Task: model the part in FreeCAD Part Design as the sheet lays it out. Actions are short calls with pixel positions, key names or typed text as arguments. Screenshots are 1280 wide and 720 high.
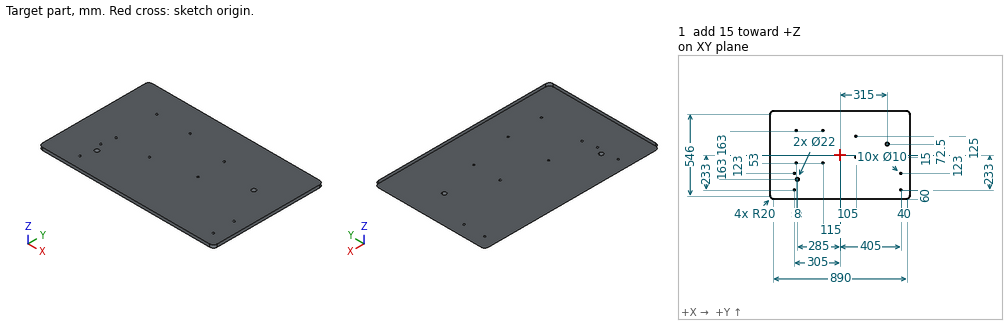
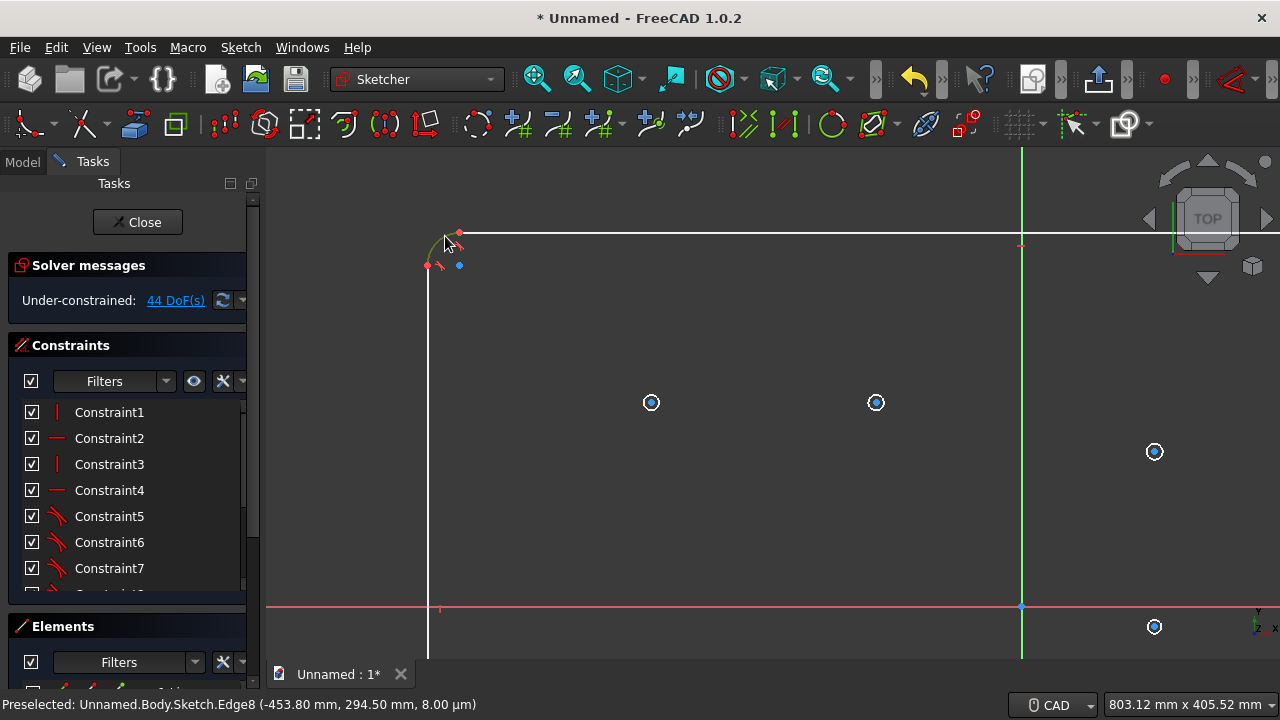
key(e)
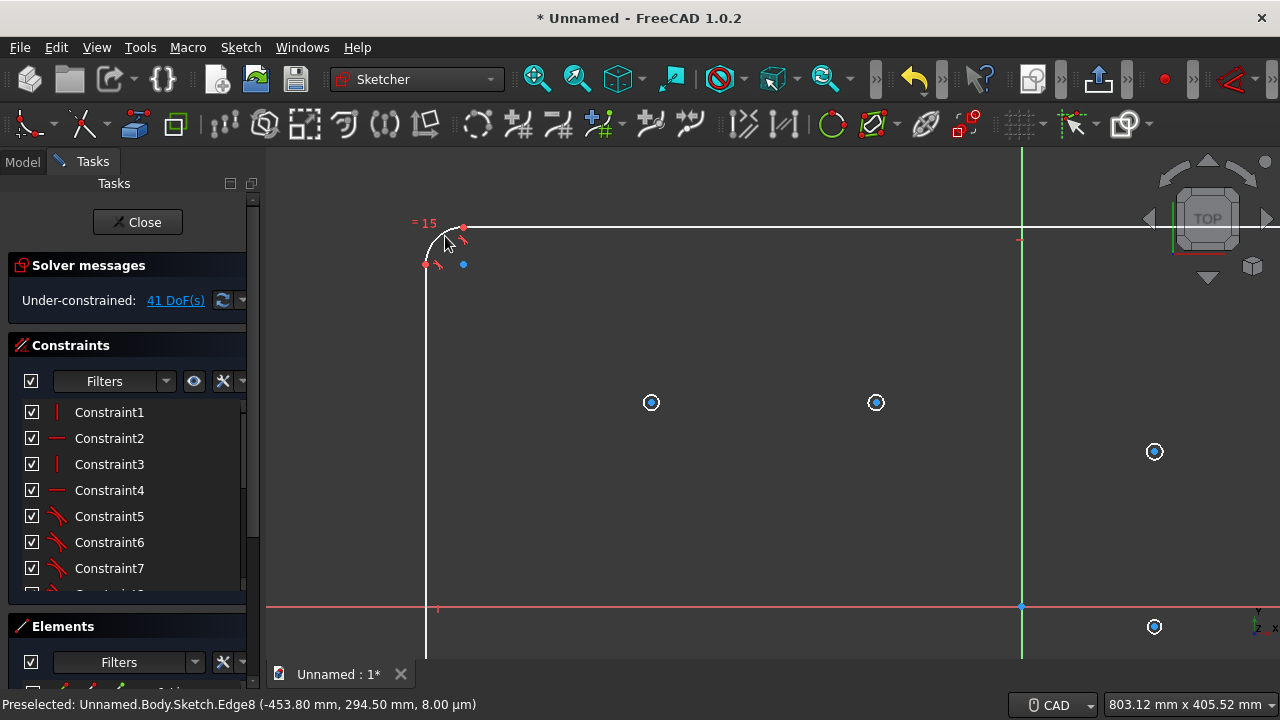
scroll(446, 237, down, 4)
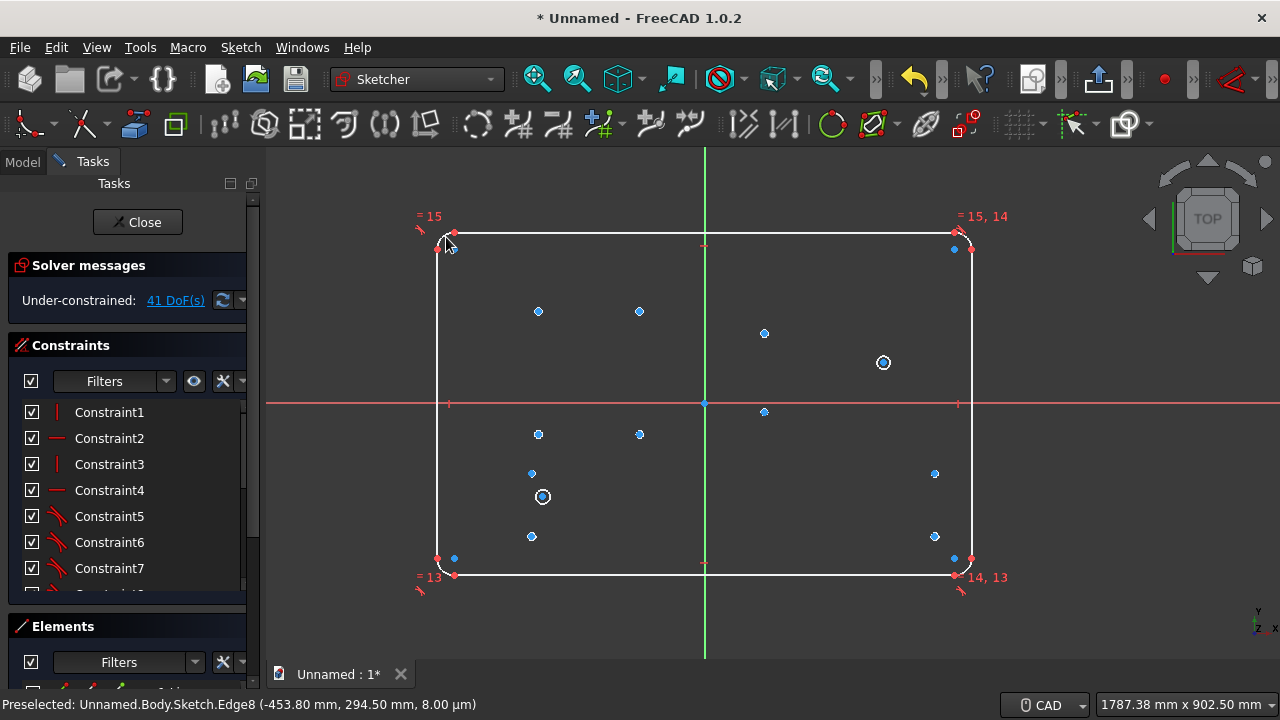
scroll(938, 534, up, 7)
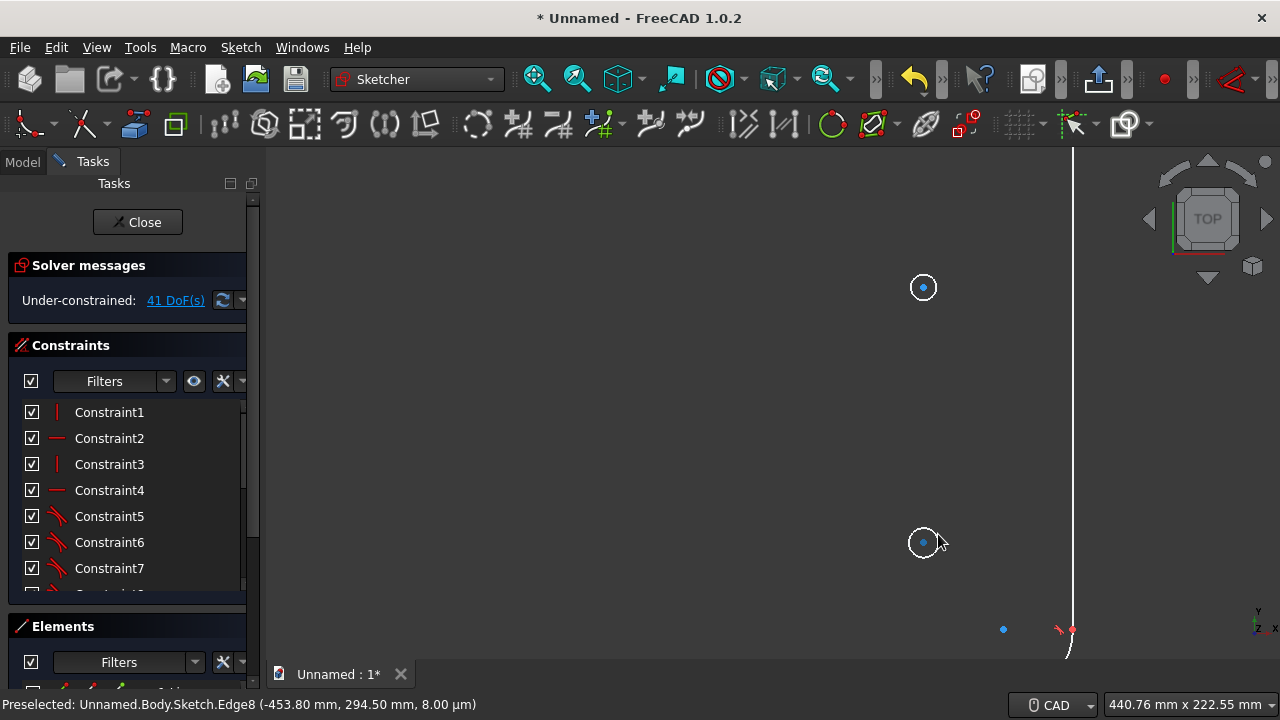
click(934, 532)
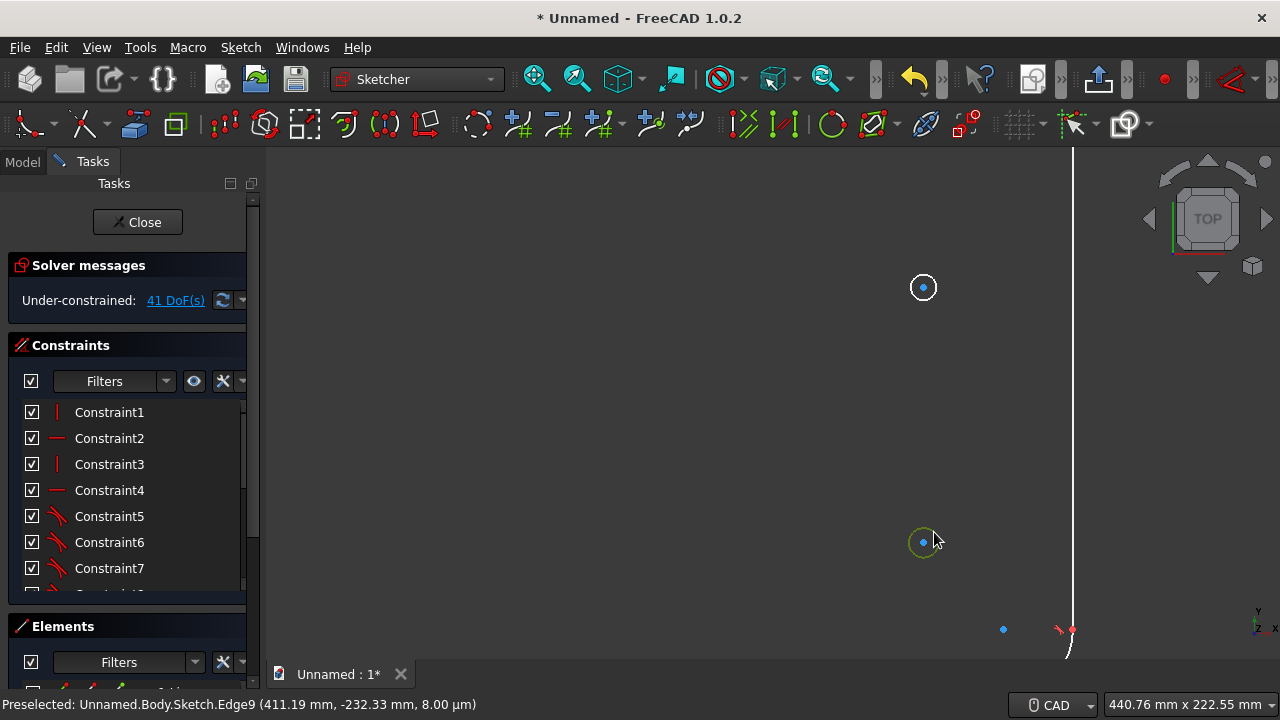
click(933, 278)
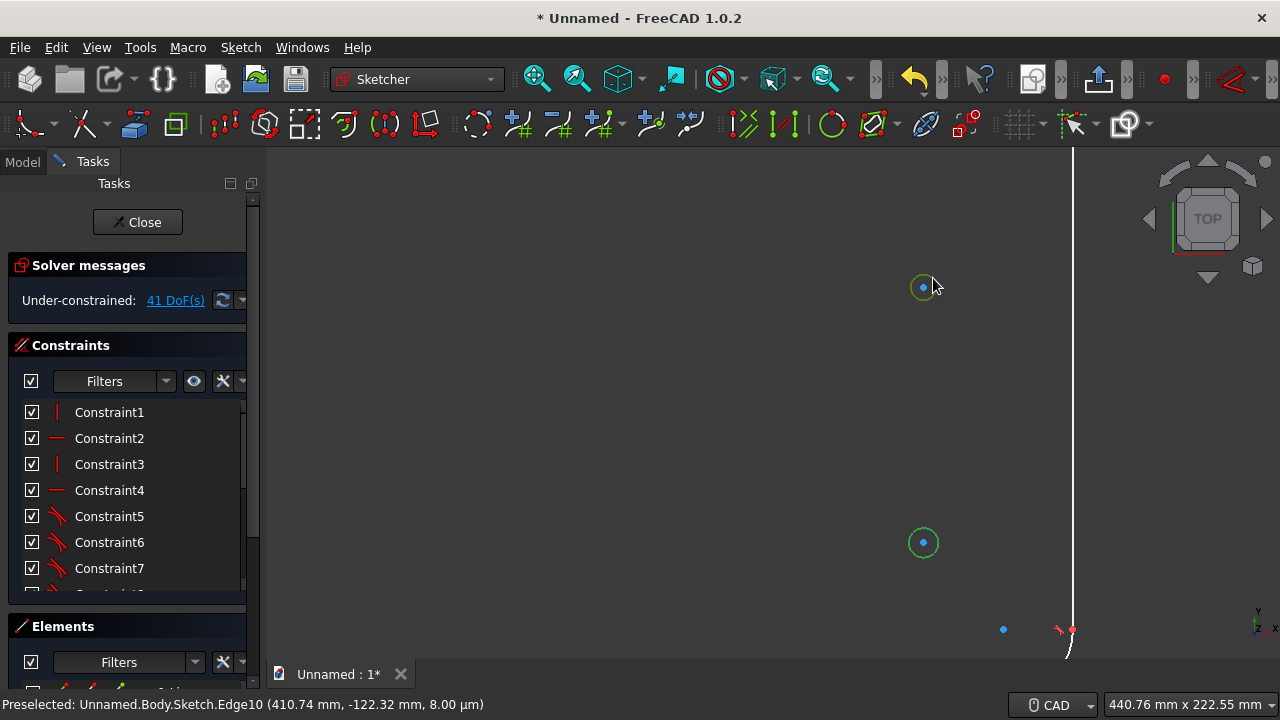
scroll(938, 534, down, 7)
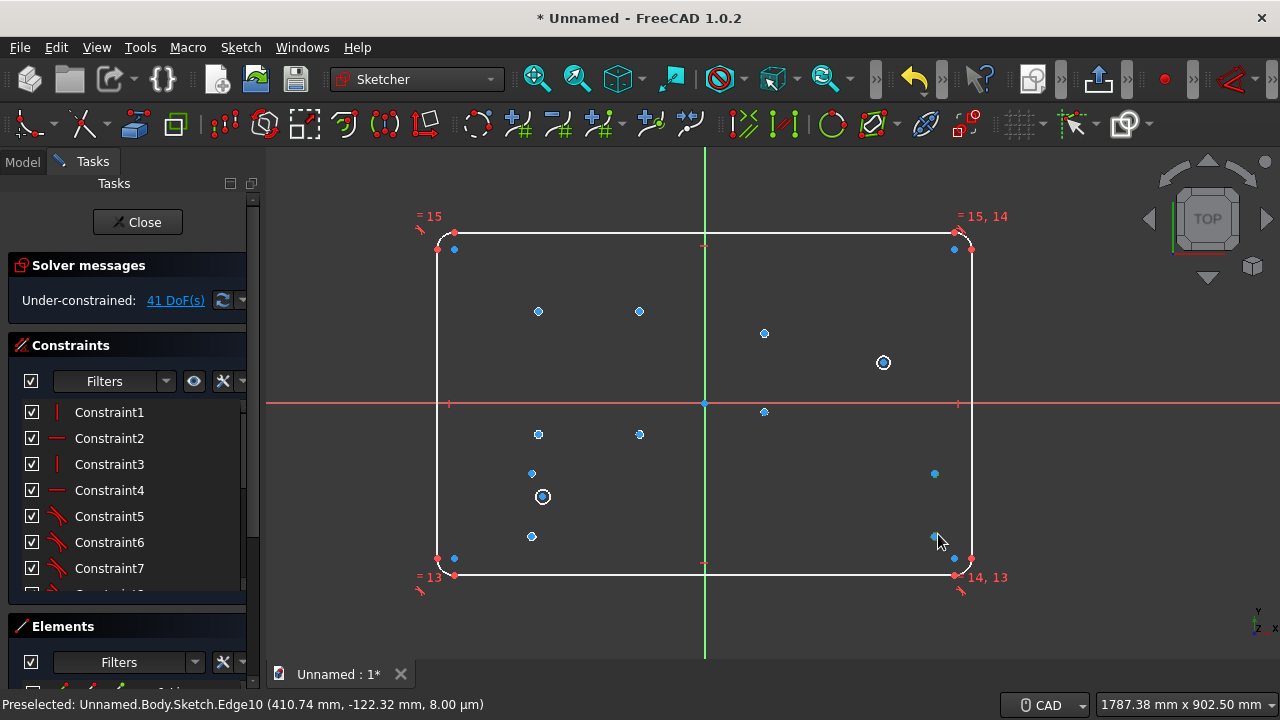
scroll(535, 534, up, 7)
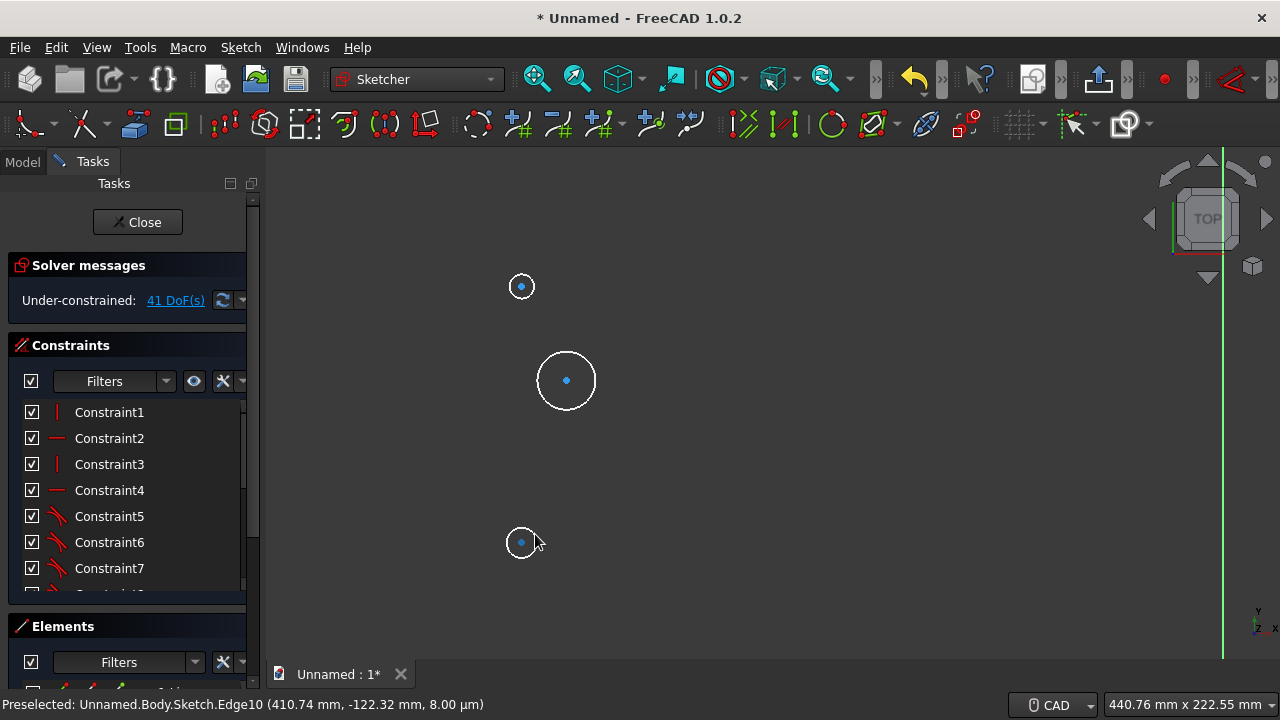
click(532, 532)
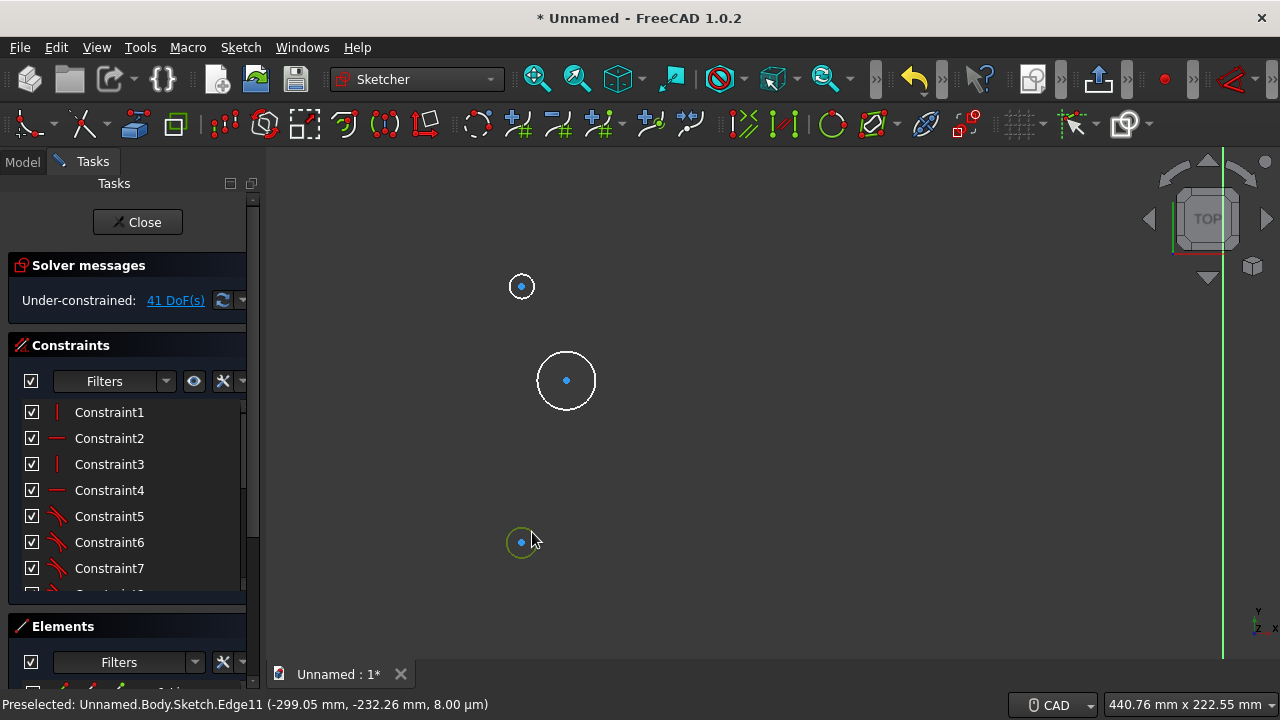
scroll(535, 534, down, 7)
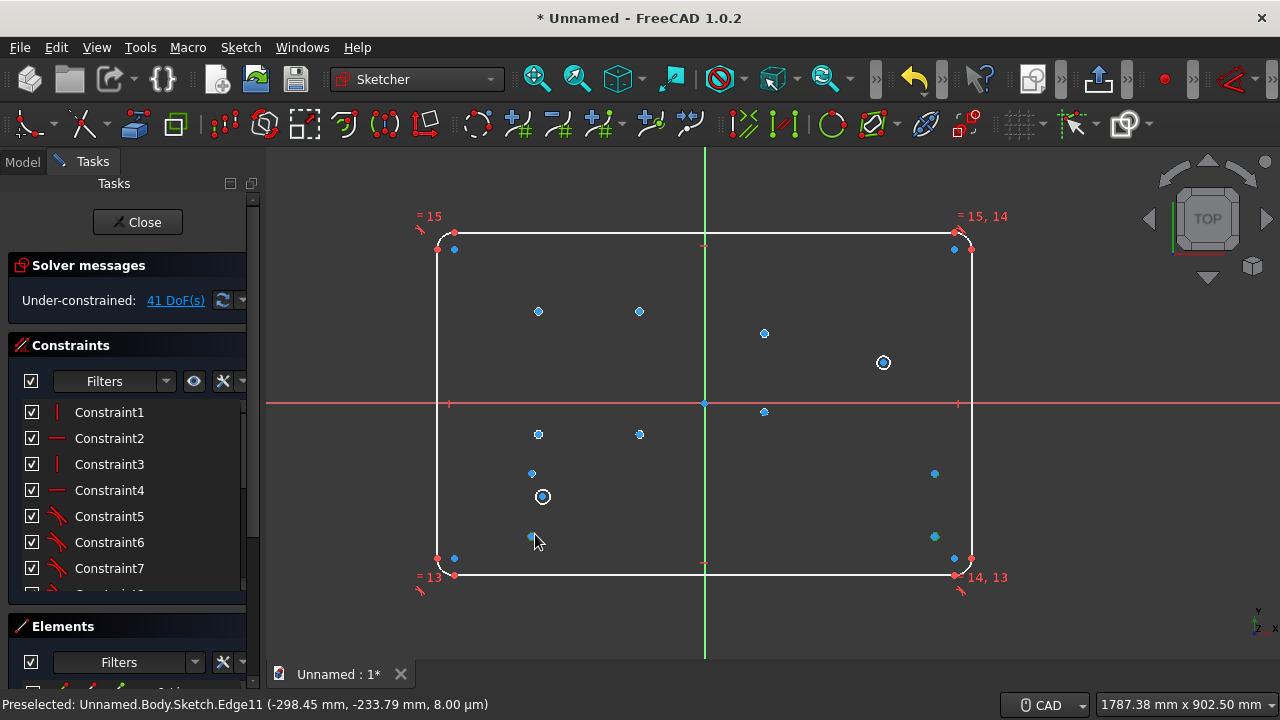
scroll(642, 432, up, 7)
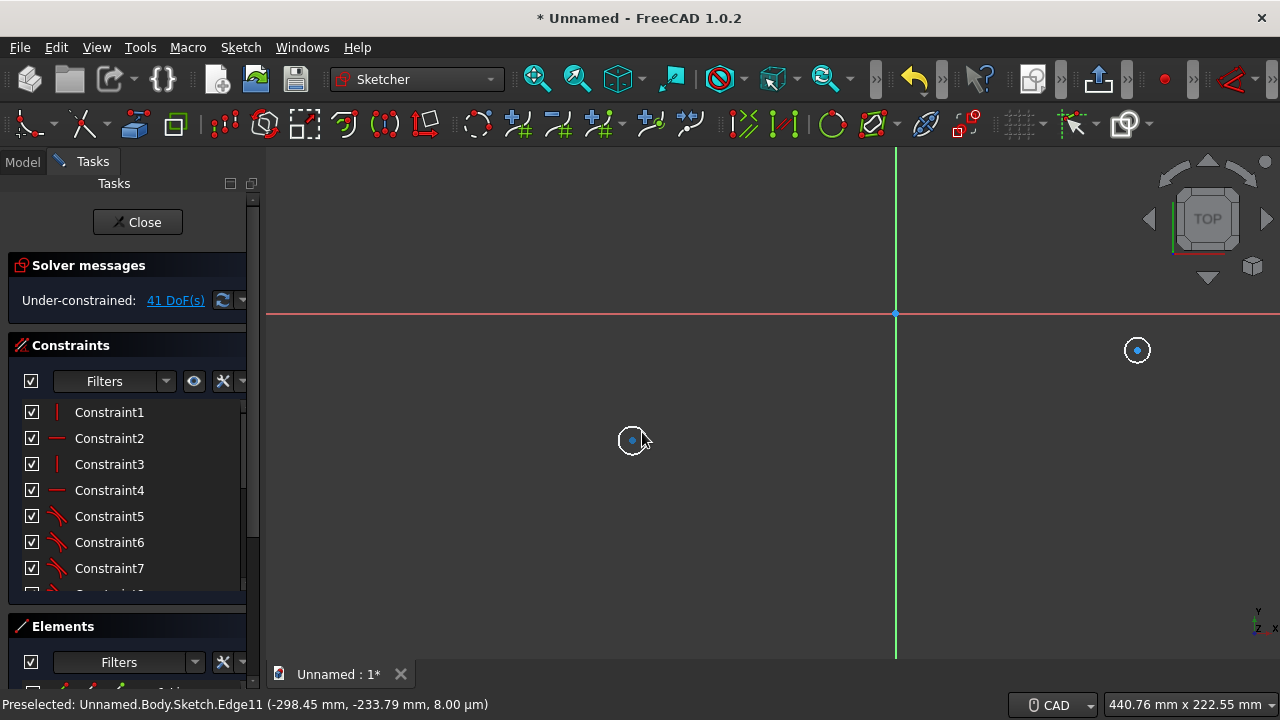
click(642, 431)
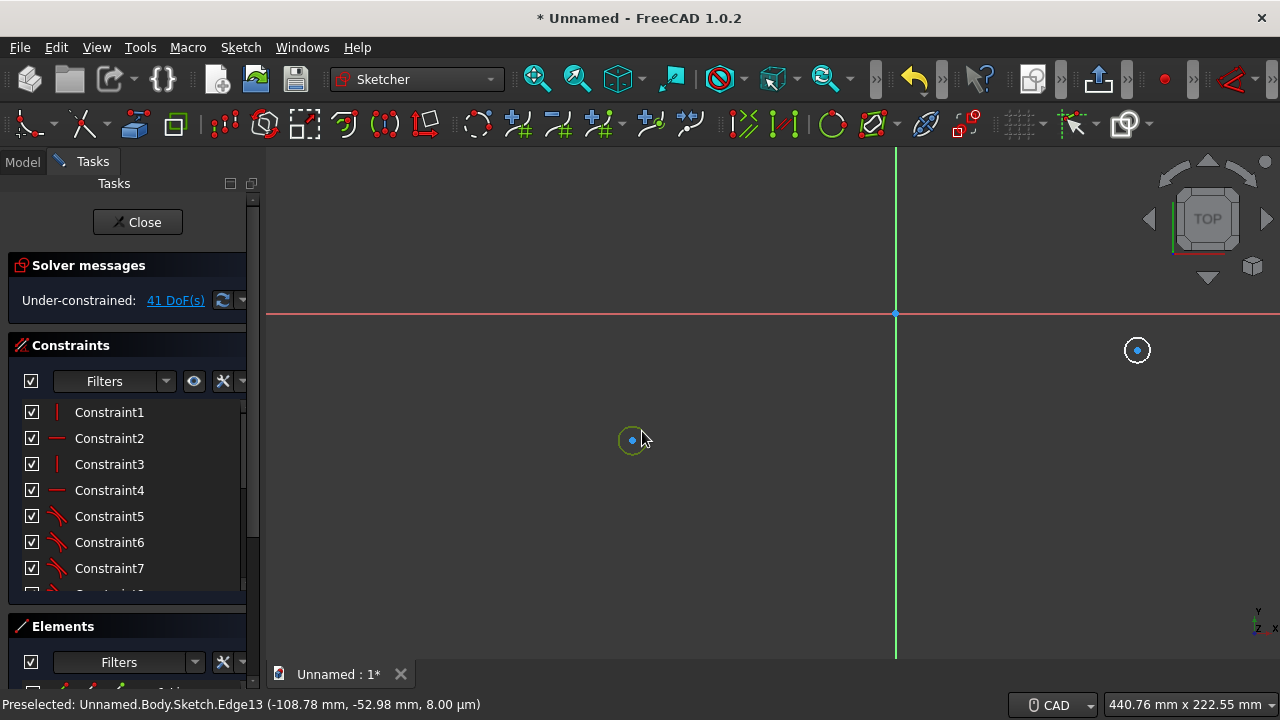
scroll(642, 432, down, 7)